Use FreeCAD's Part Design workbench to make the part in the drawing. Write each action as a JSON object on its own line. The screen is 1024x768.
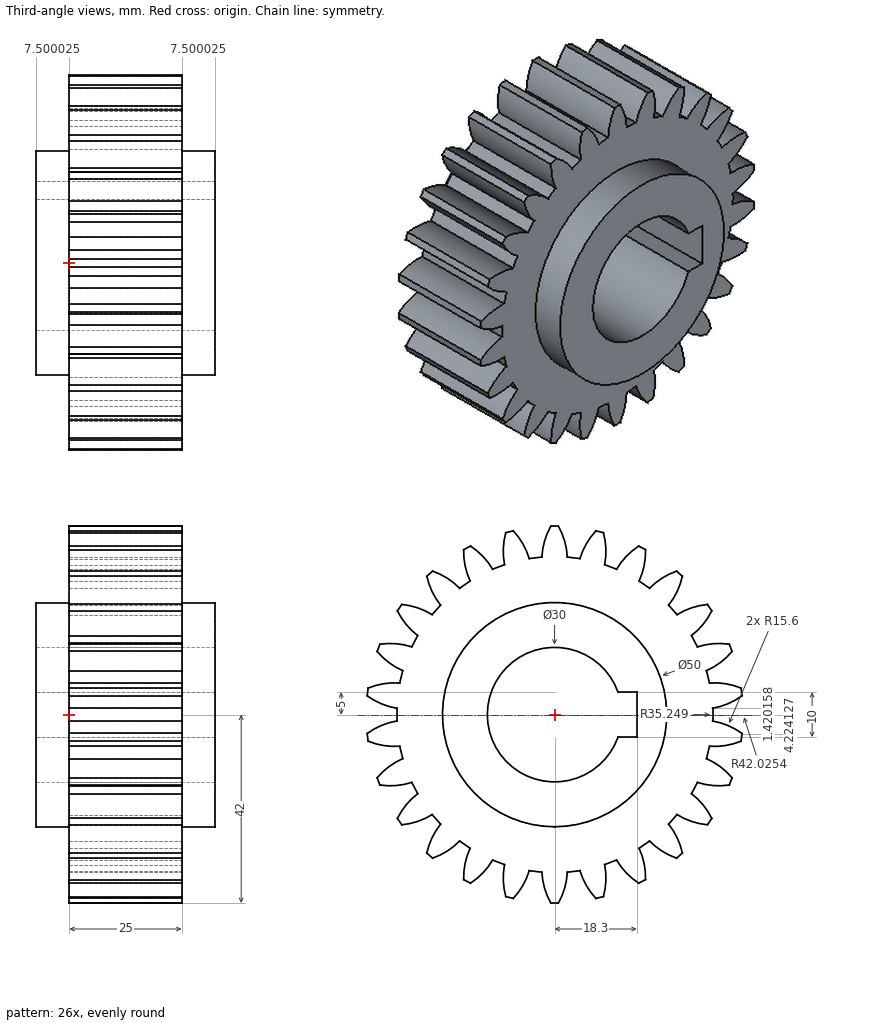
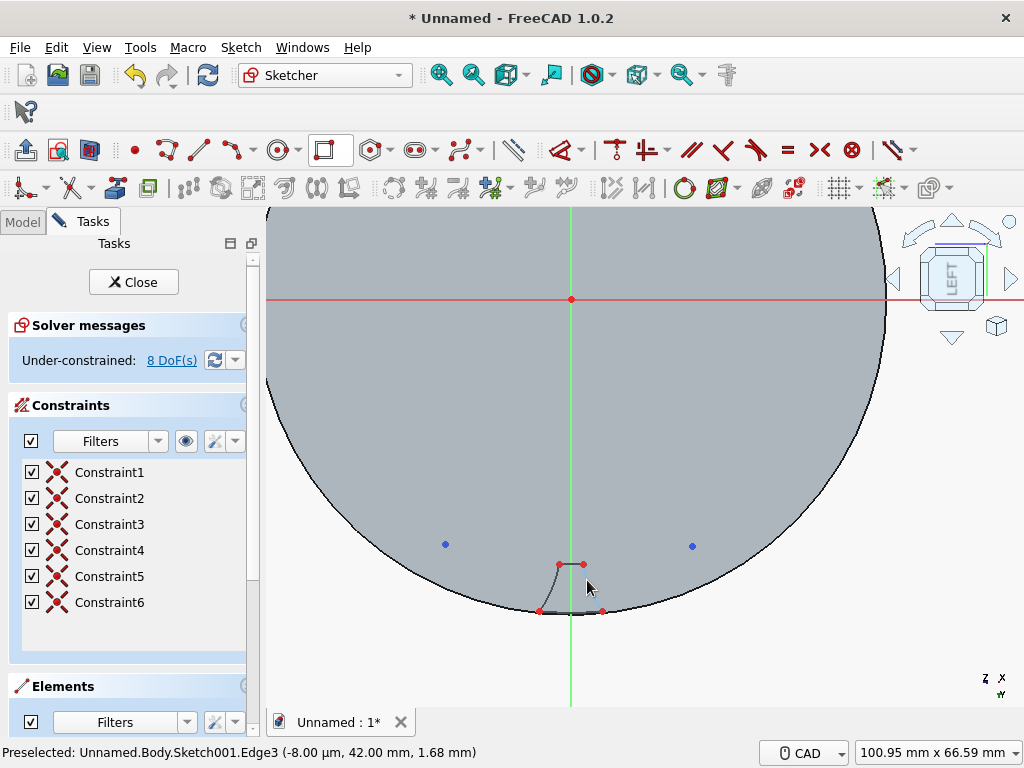
{"action": "left_click", "coordinate": [587, 579]}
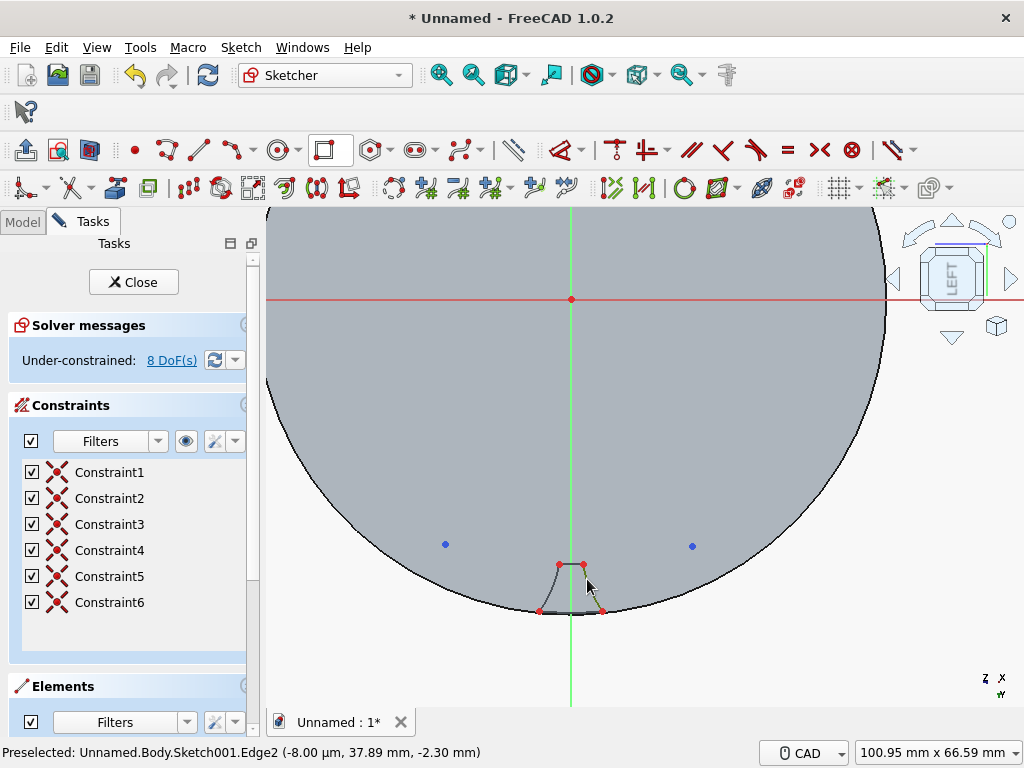
{"action": "left_click", "coordinate": [548, 598]}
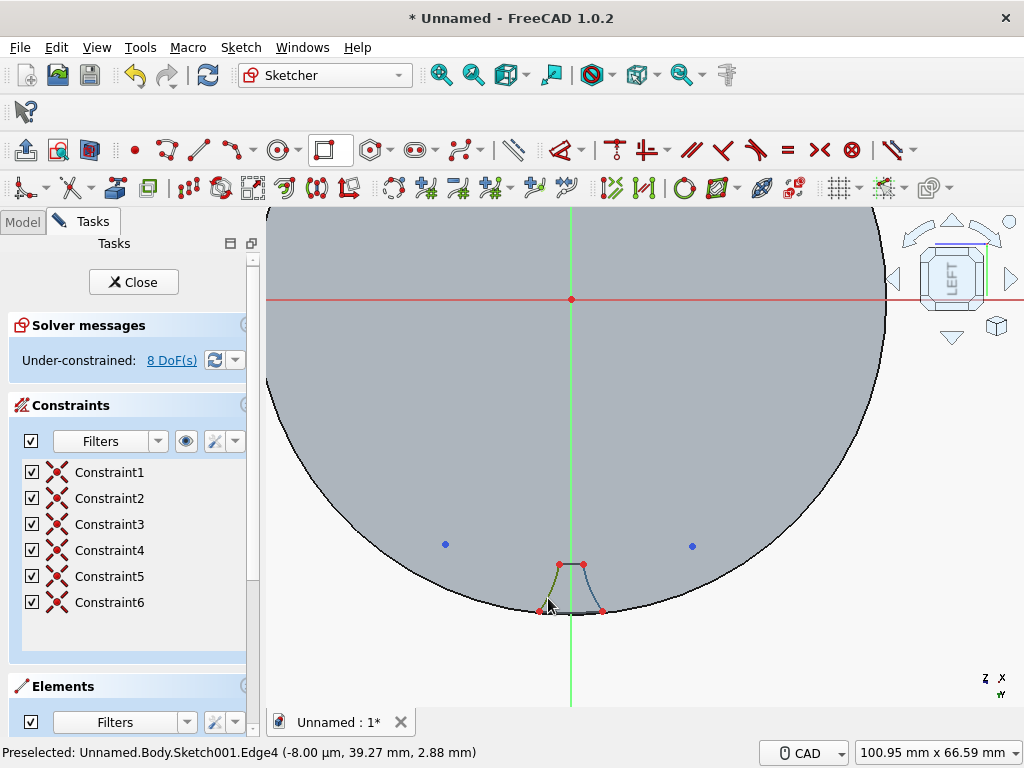
{"action": "left_click", "coordinate": [788, 150]}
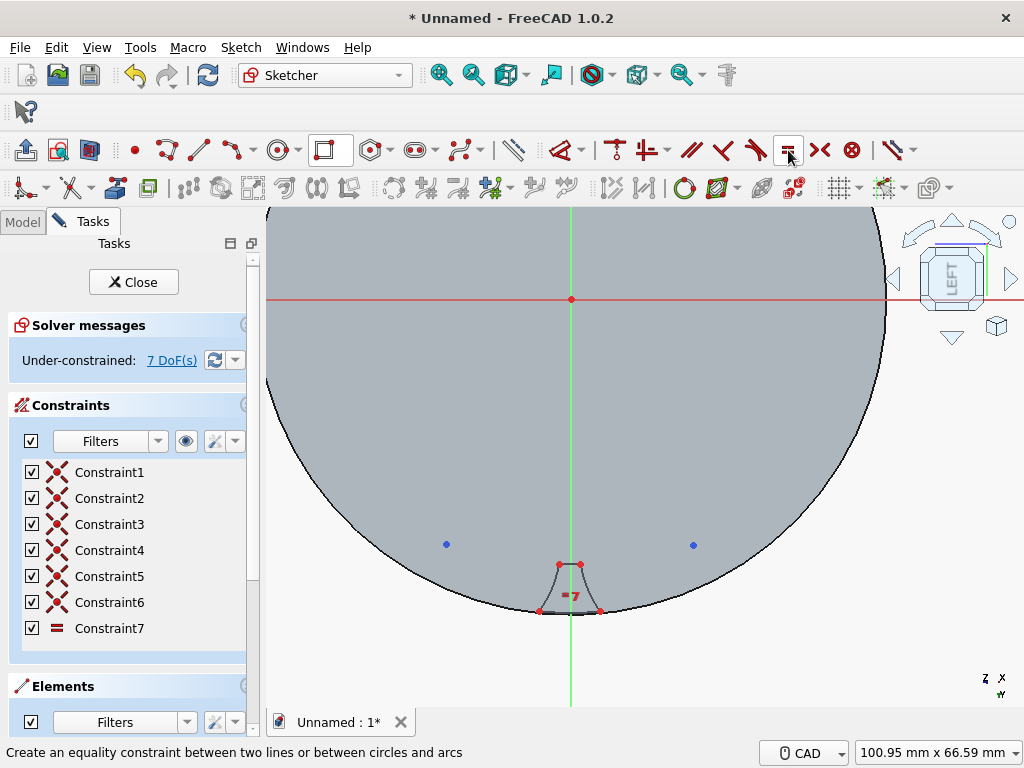
{"action": "left_click", "coordinate": [693, 546]}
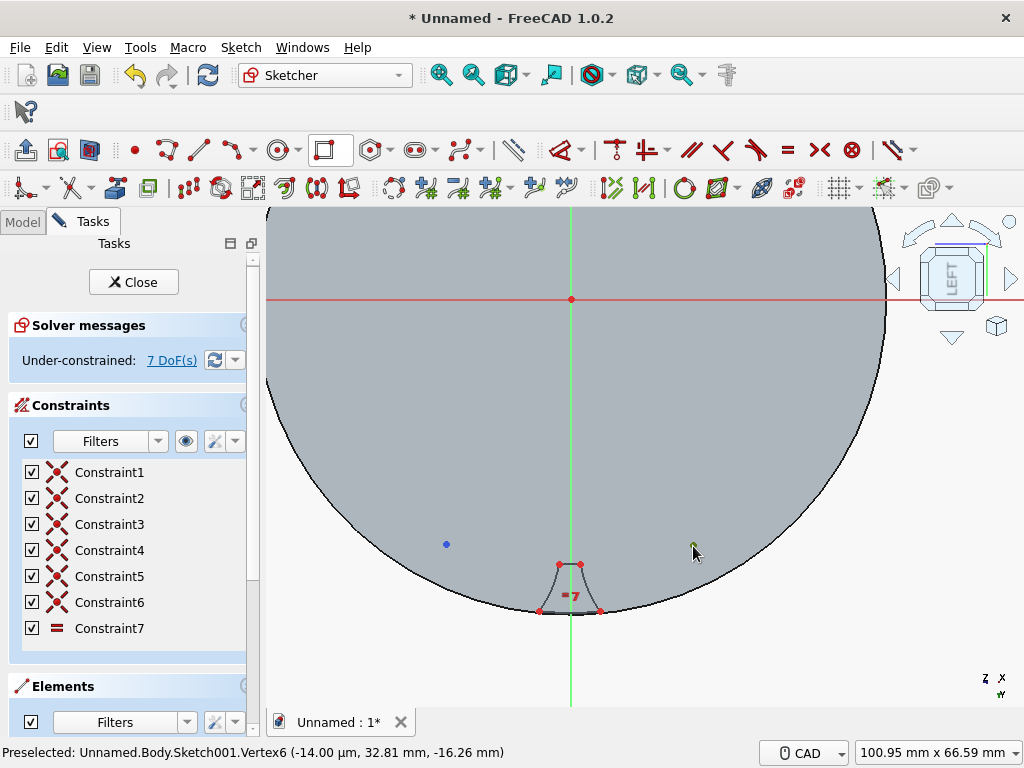
{"action": "left_click", "coordinate": [447, 544]}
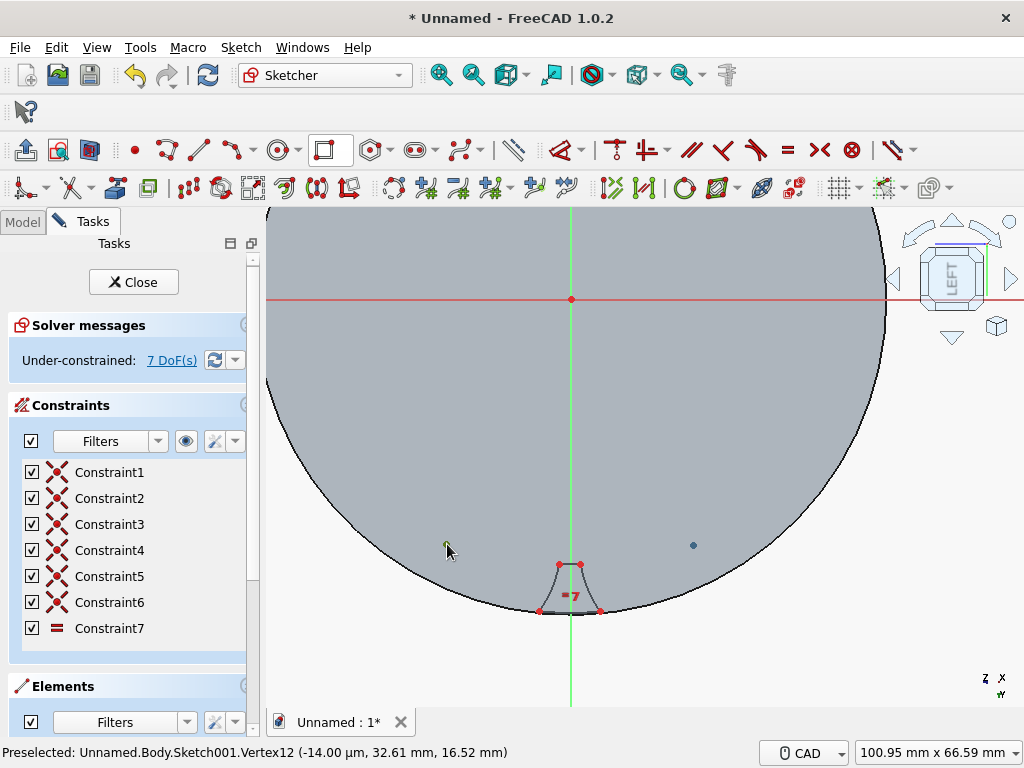
{"action": "left_click", "coordinate": [571, 647]}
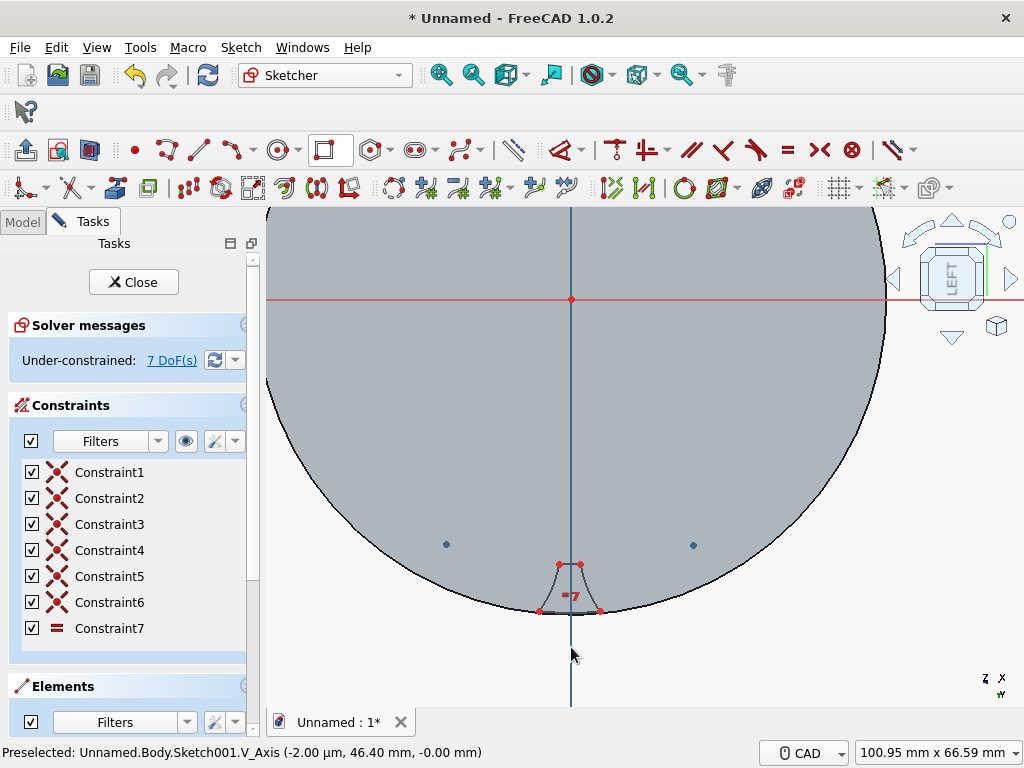
{"action": "left_click", "coordinate": [820, 150]}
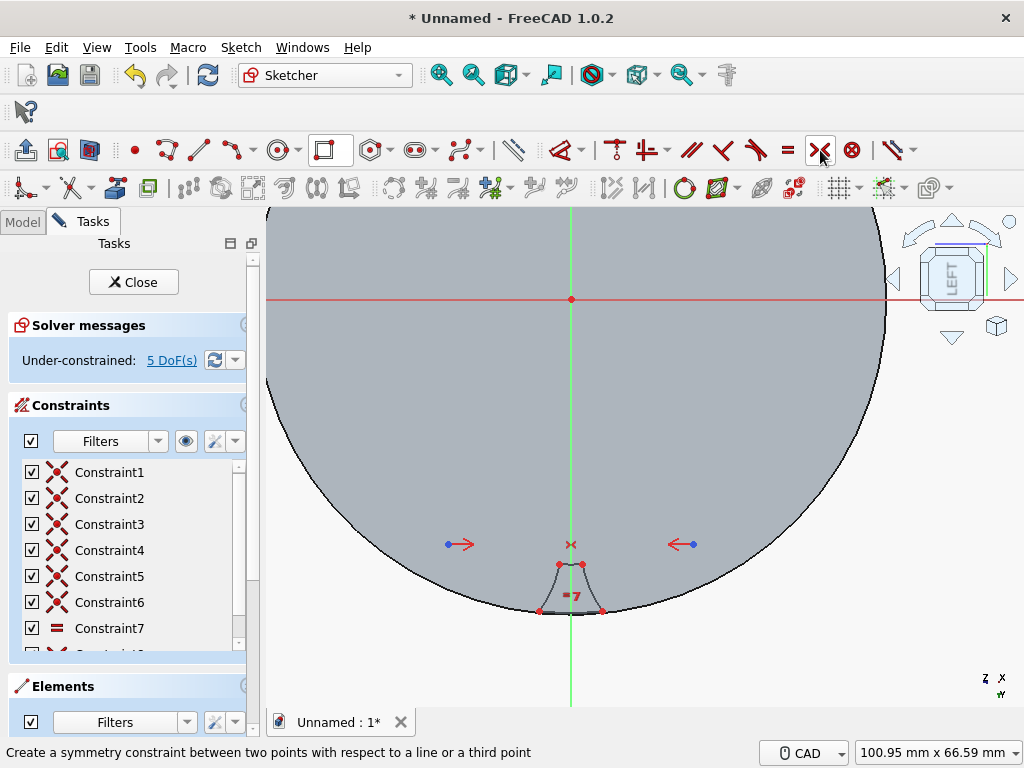
{"action": "left_click", "coordinate": [560, 150]}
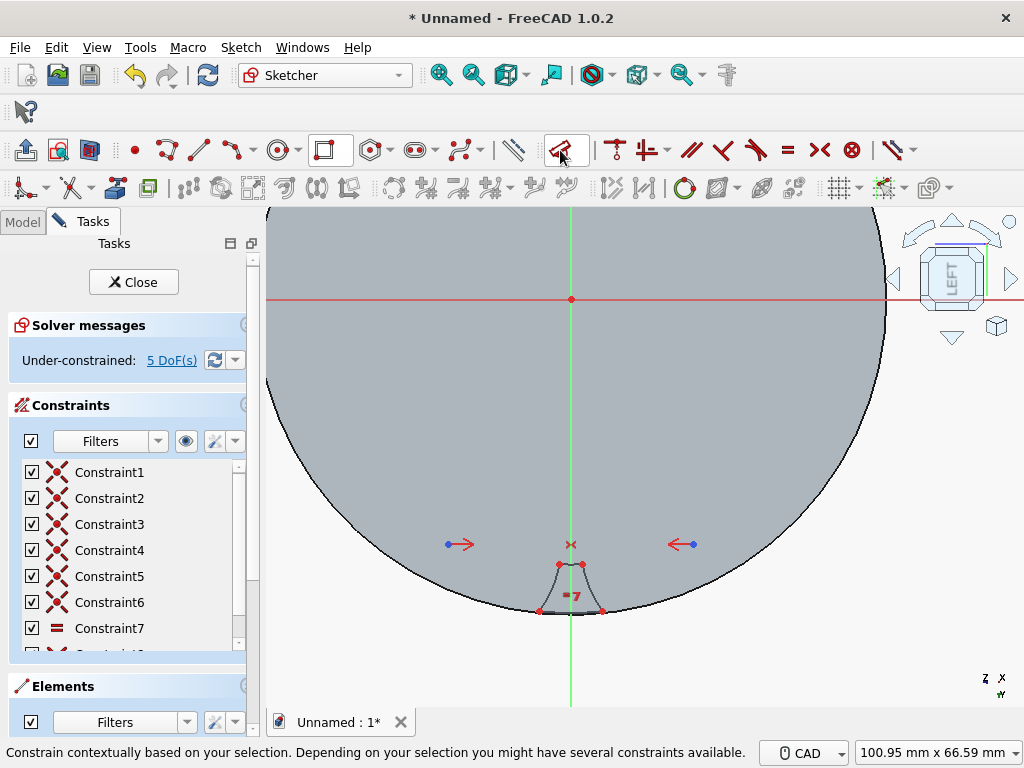
{"action": "left_click", "coordinate": [571, 565]}
{"action": "left_click", "coordinate": [428, 561]}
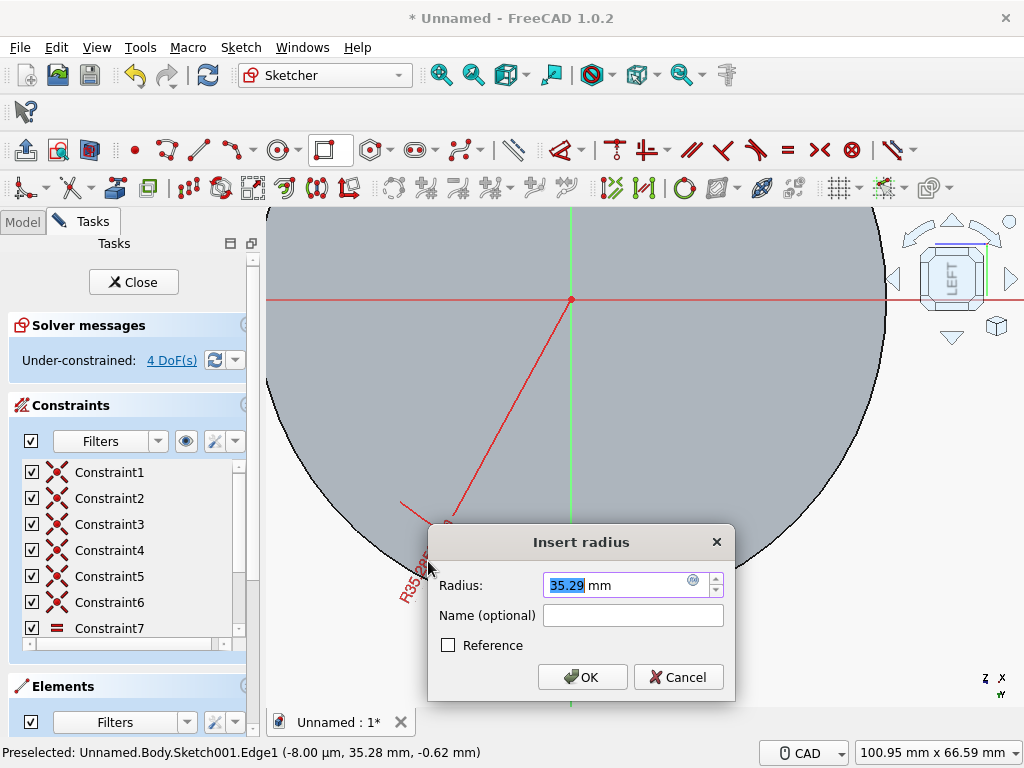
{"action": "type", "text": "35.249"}
{"action": "key", "text": "Return"}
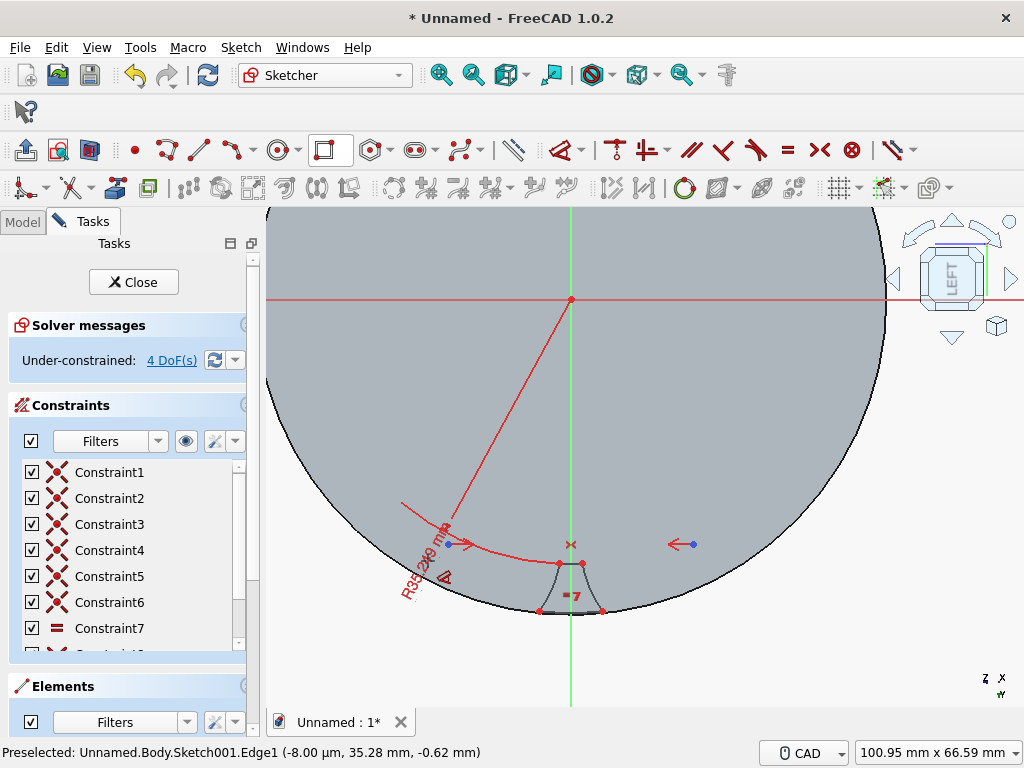
{"action": "left_click", "coordinate": [586, 579]}
{"action": "left_click", "coordinate": [551, 517]}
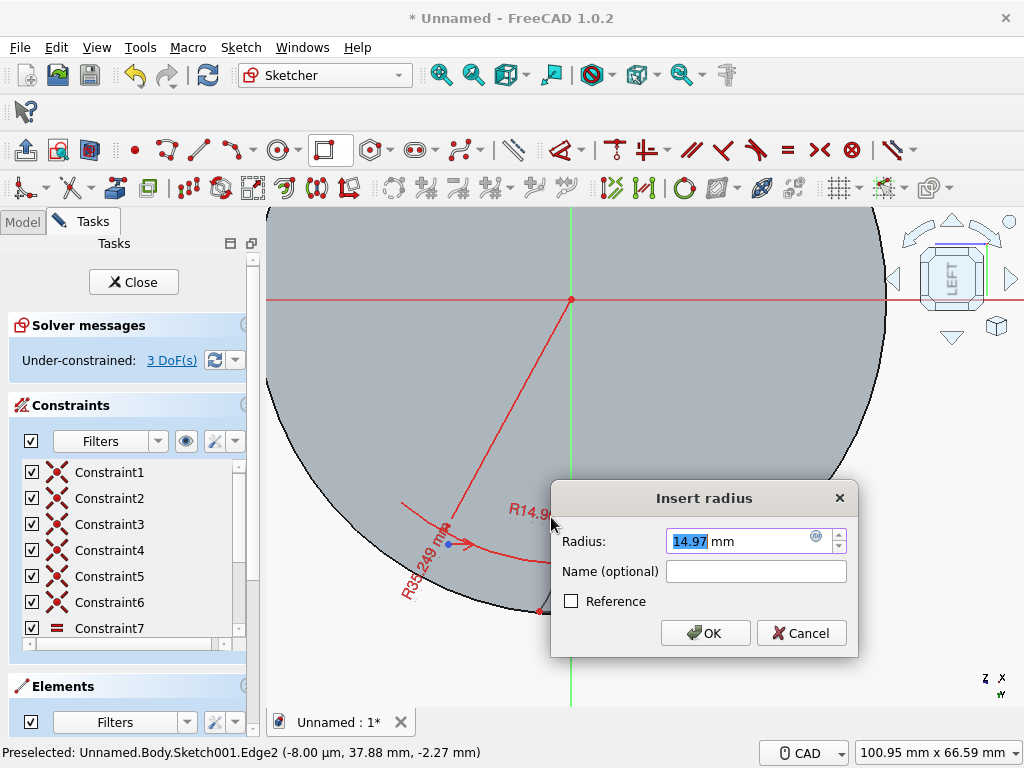
{"action": "type", "text": "15.6"}
{"action": "key", "text": "Return"}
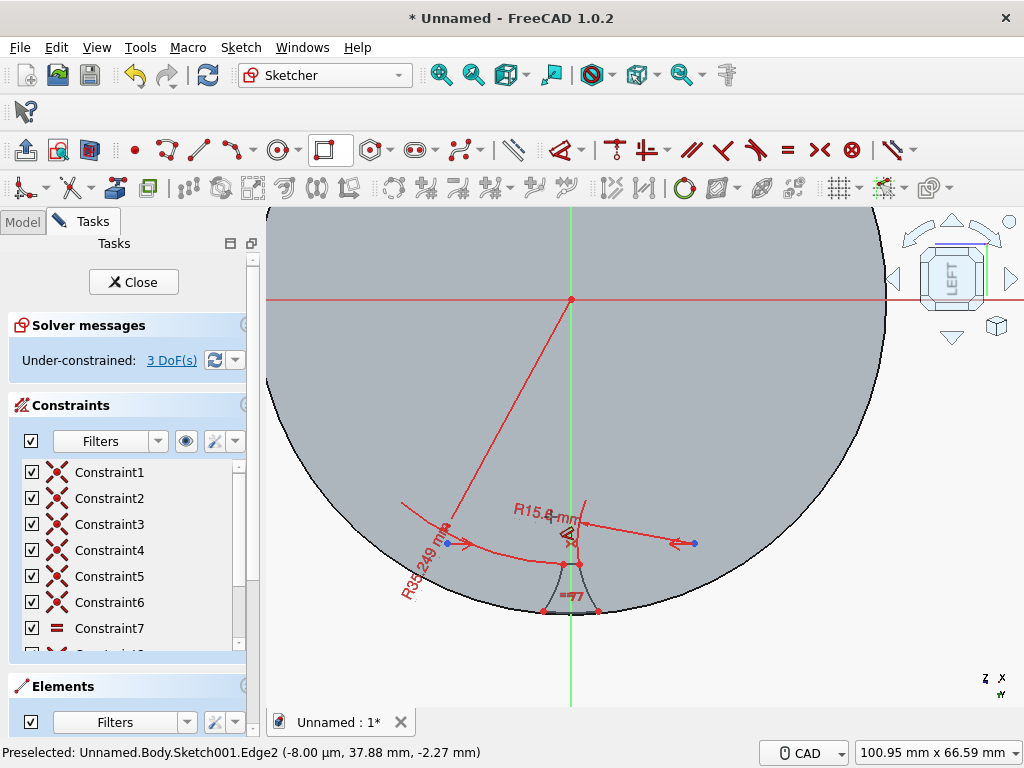
{"action": "scroll", "coordinate": [560, 613], "scroll_direction": "up", "scroll_amount": 2}